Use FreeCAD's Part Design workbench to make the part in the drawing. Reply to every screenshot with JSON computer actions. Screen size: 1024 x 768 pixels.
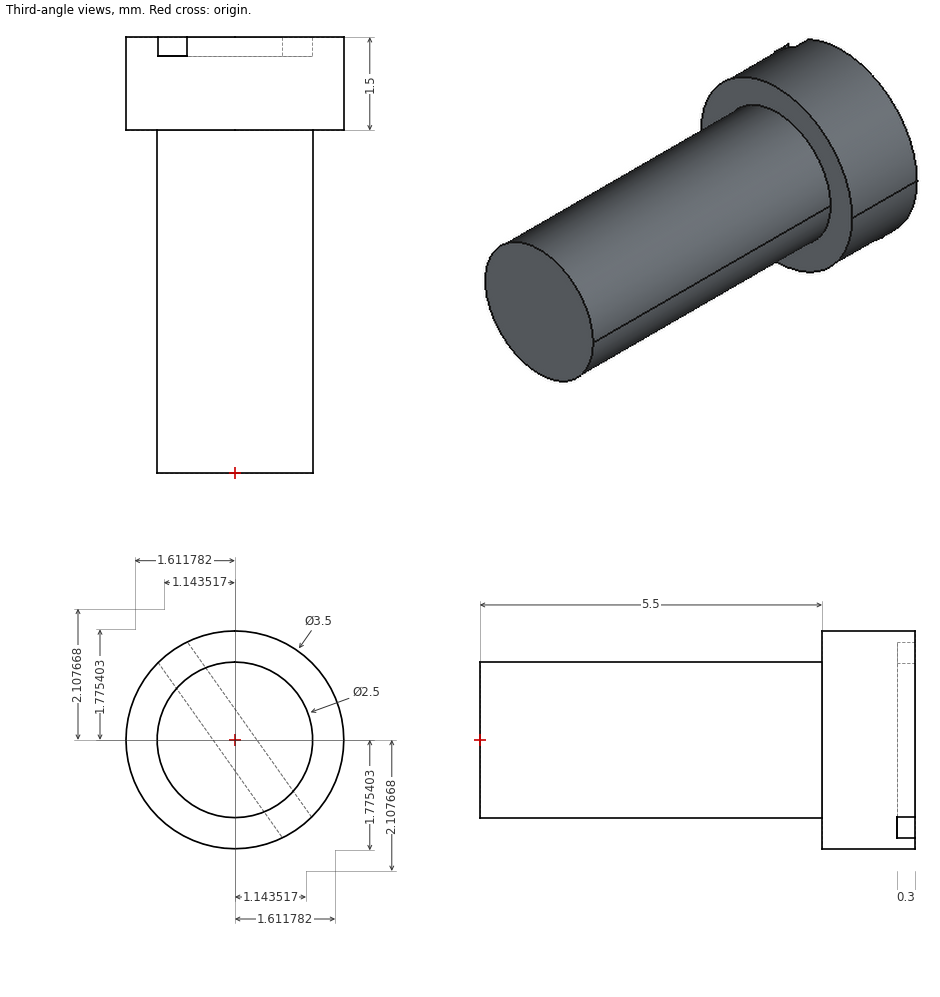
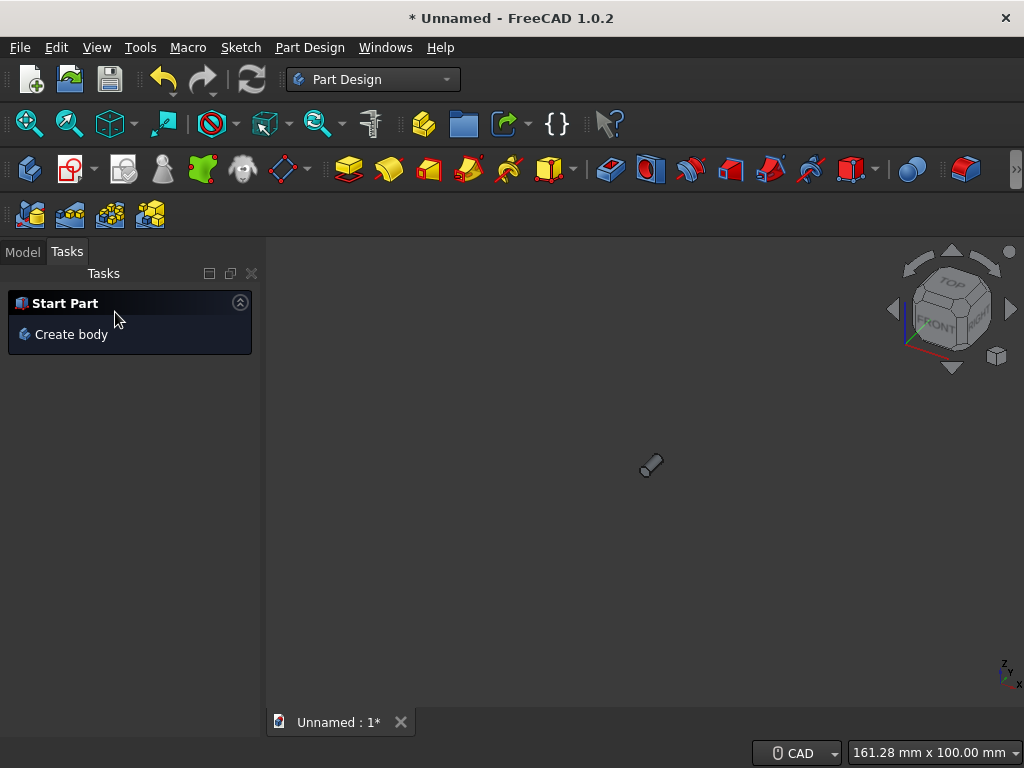
{"action": "key", "text": "v f"}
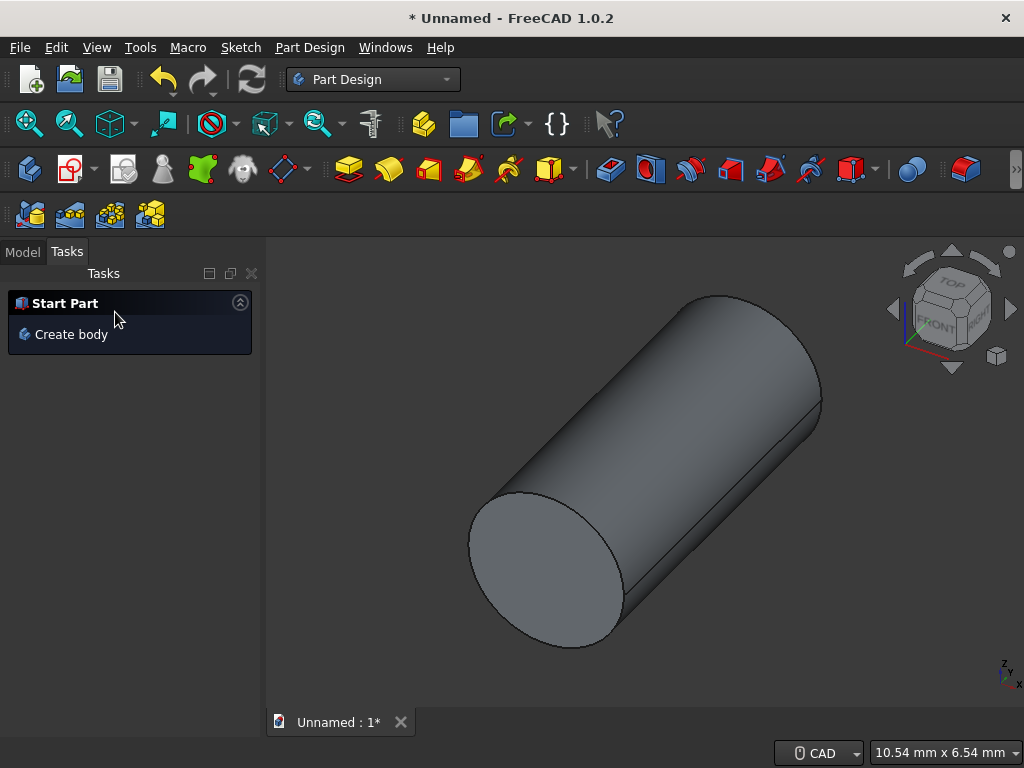
{"action": "key", "text": "4"}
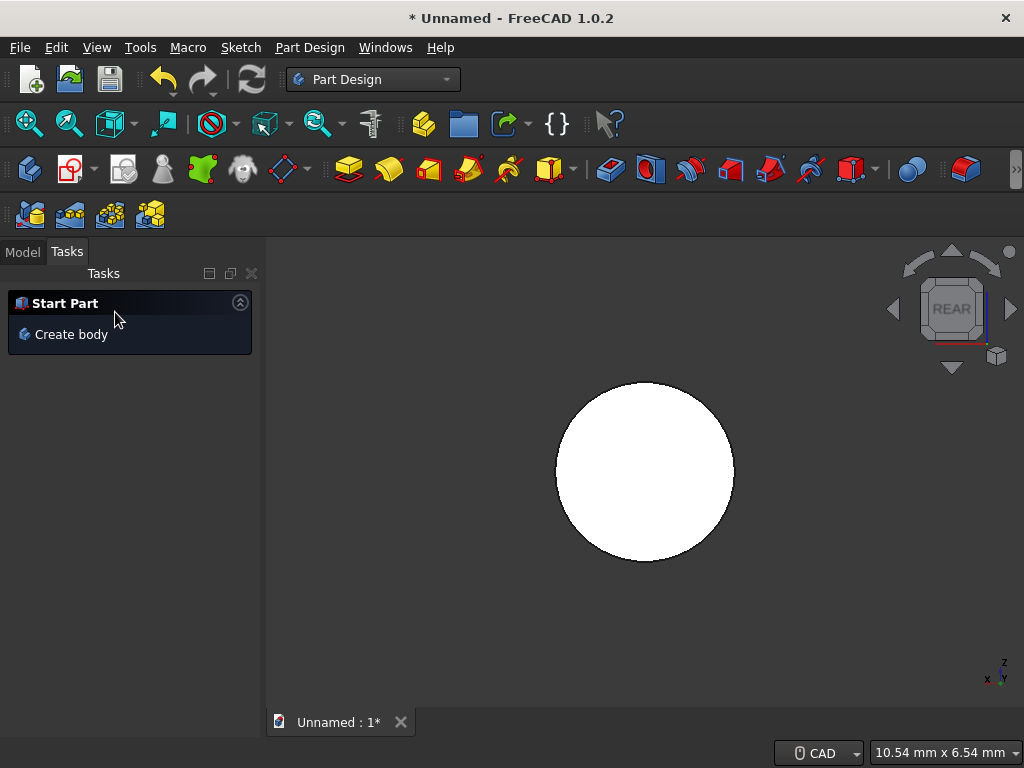
{"action": "left_click", "coordinate": [30, 124]}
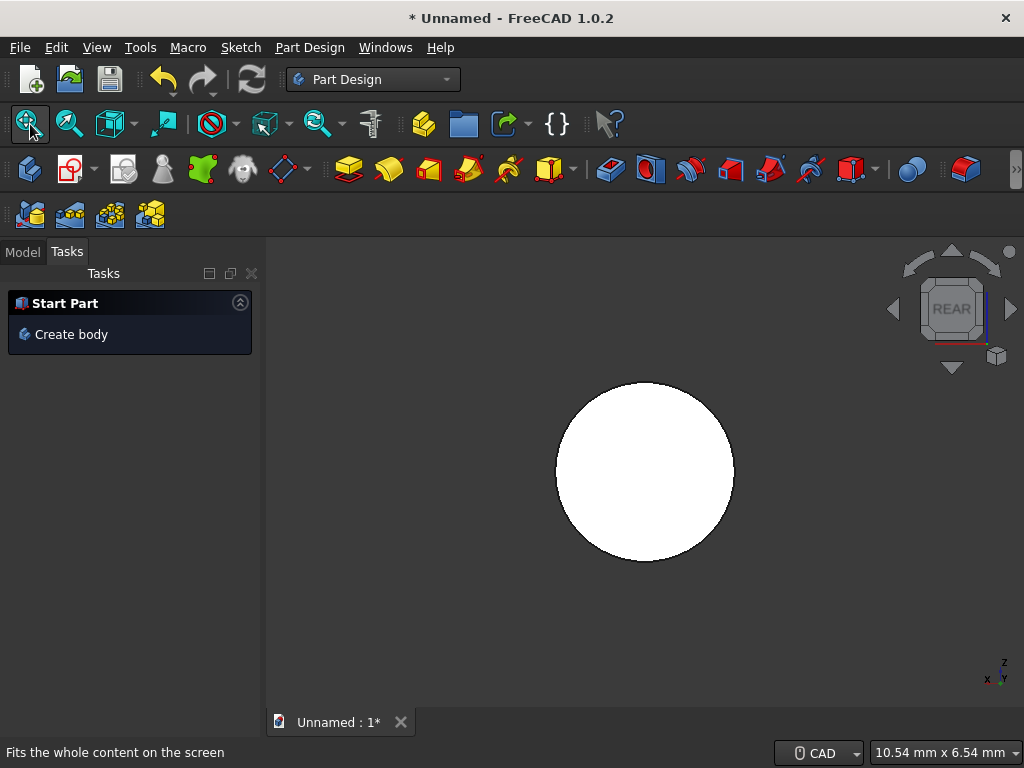
{"action": "left_click", "coordinate": [645, 471]}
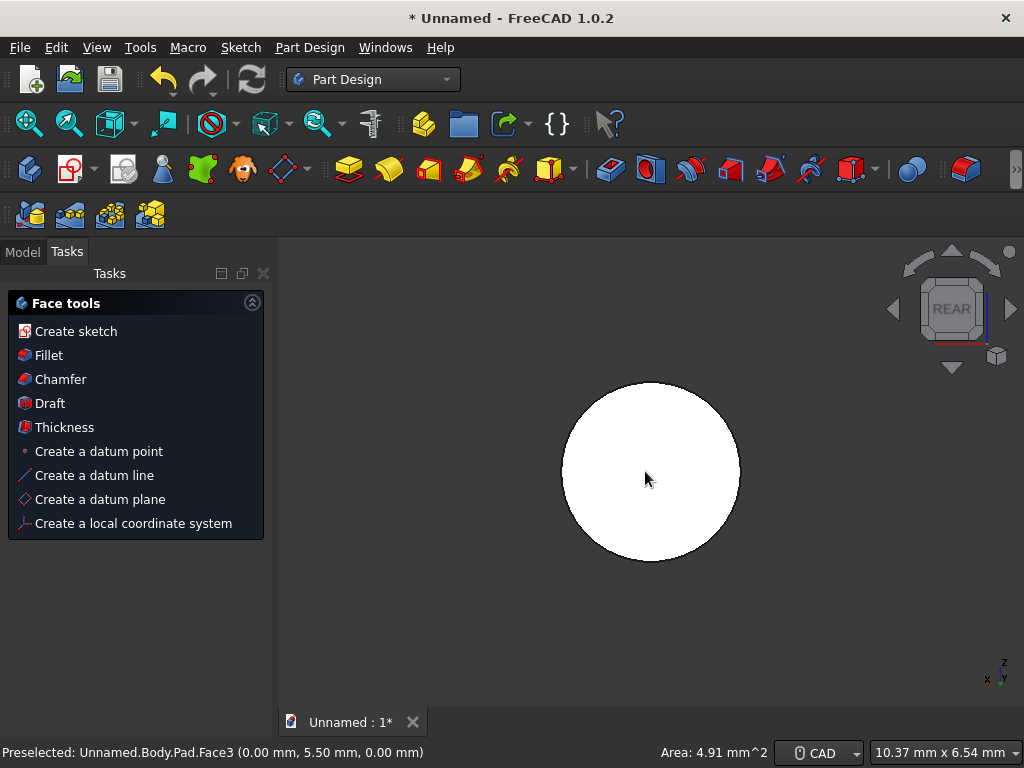
{"action": "left_click", "coordinate": [70, 170]}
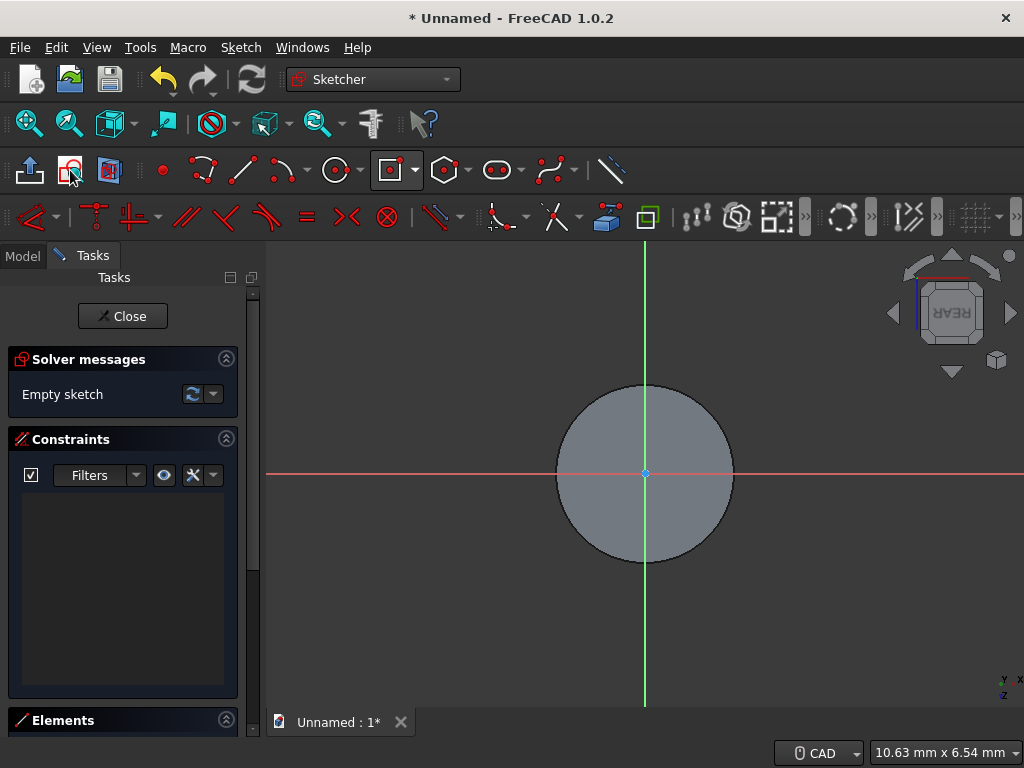
{"action": "key", "text": "g c"}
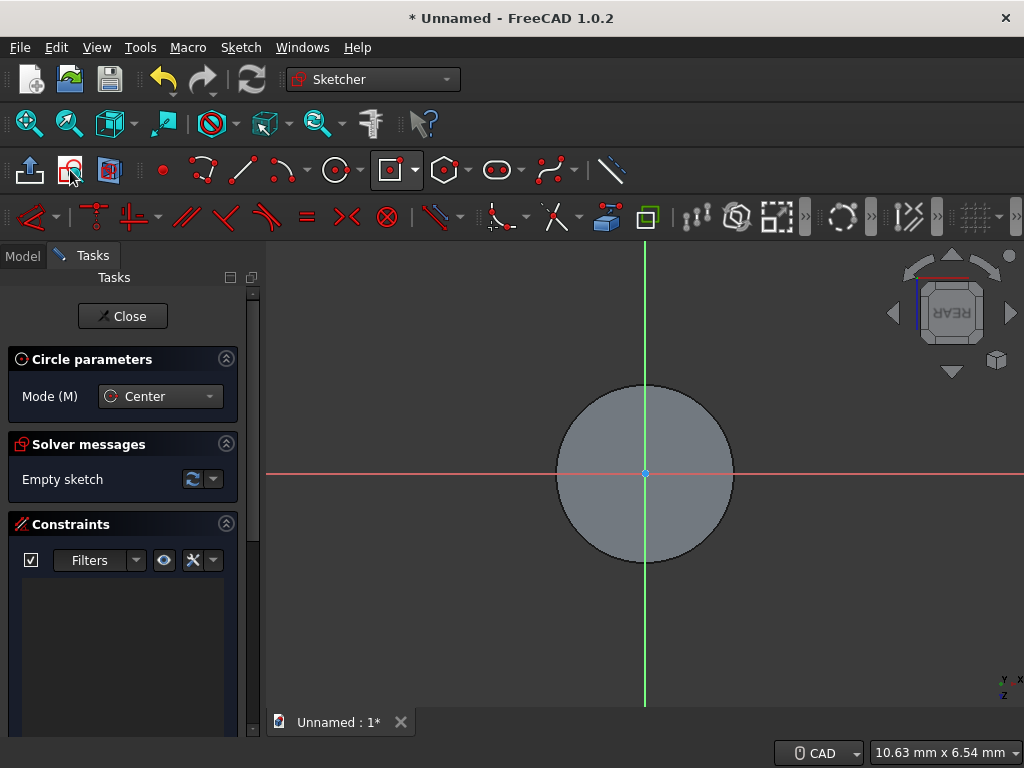
{"action": "left_click", "coordinate": [645, 474]}
{"action": "mouse_move", "coordinate": [733, 386]}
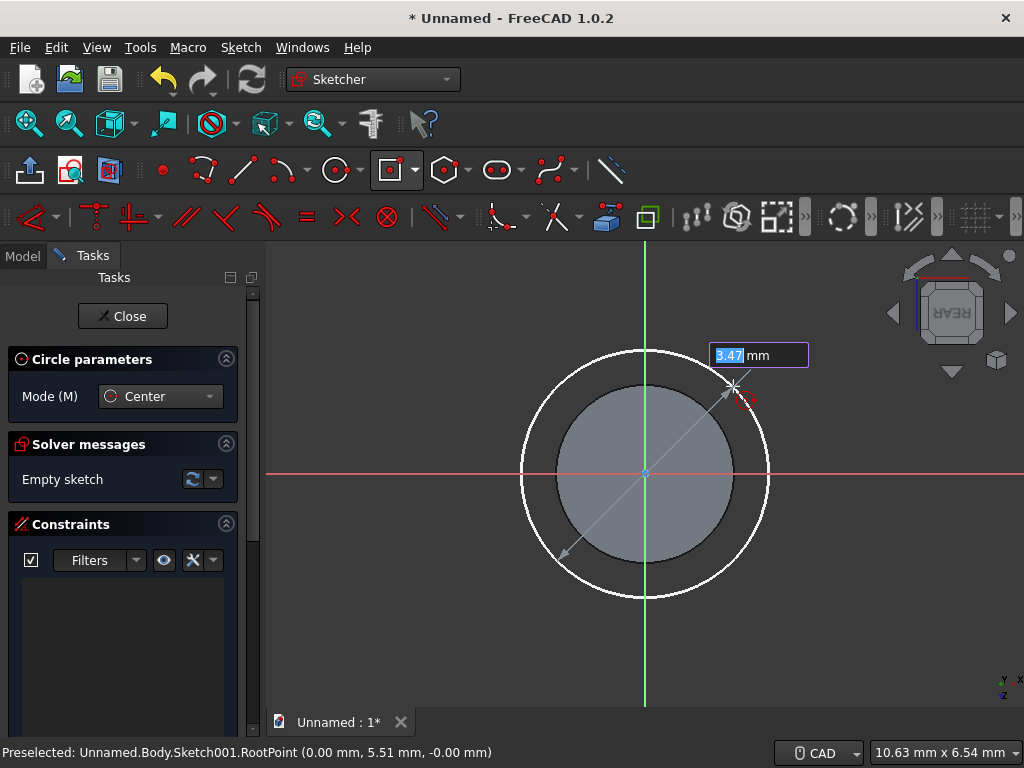
{"action": "type", "text": "3.5"}
{"action": "key", "text": "Return"}
{"action": "key", "text": "Escape"}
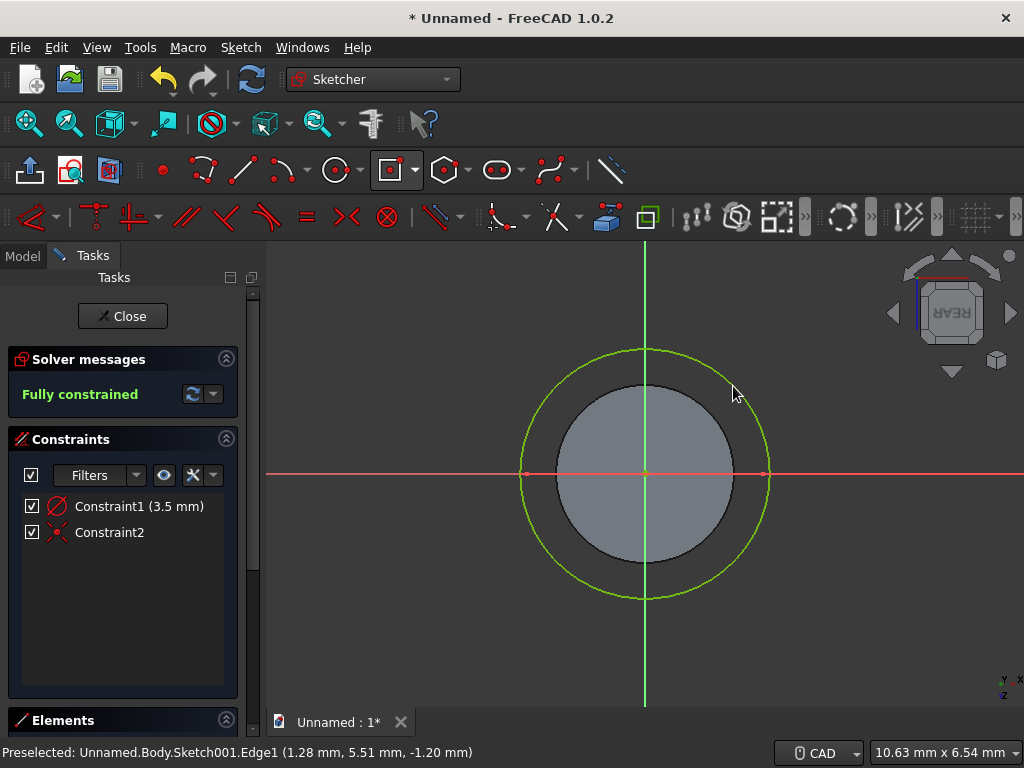
{"action": "left_click", "coordinate": [123, 316]}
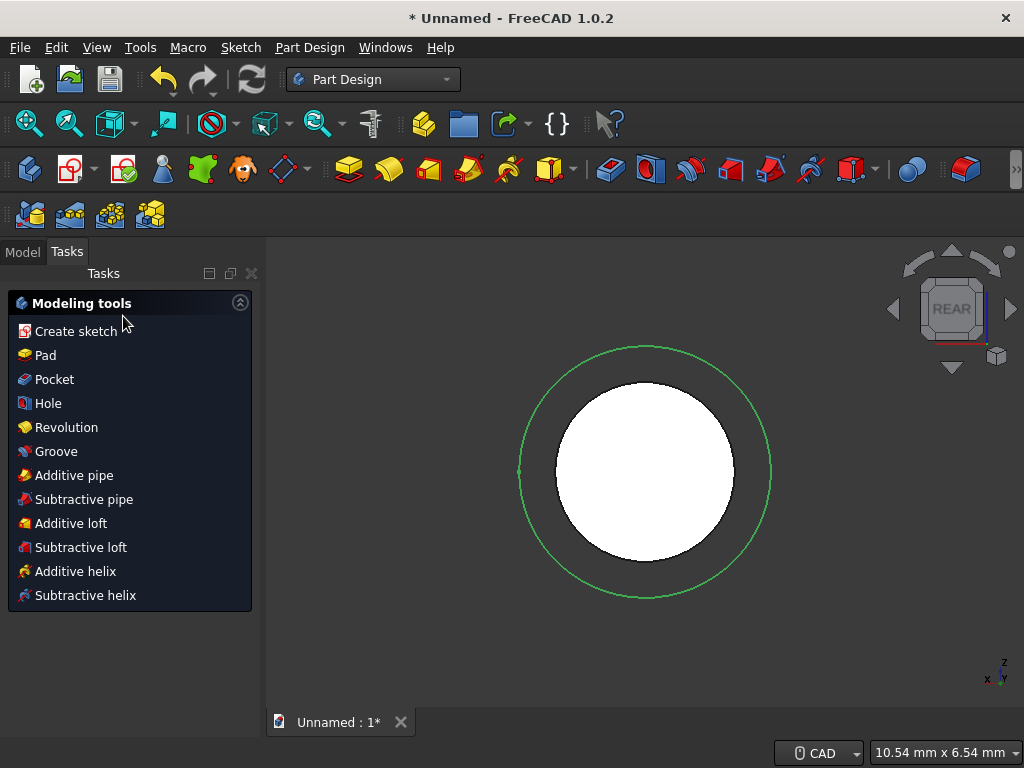
{"action": "left_click", "coordinate": [350, 170]}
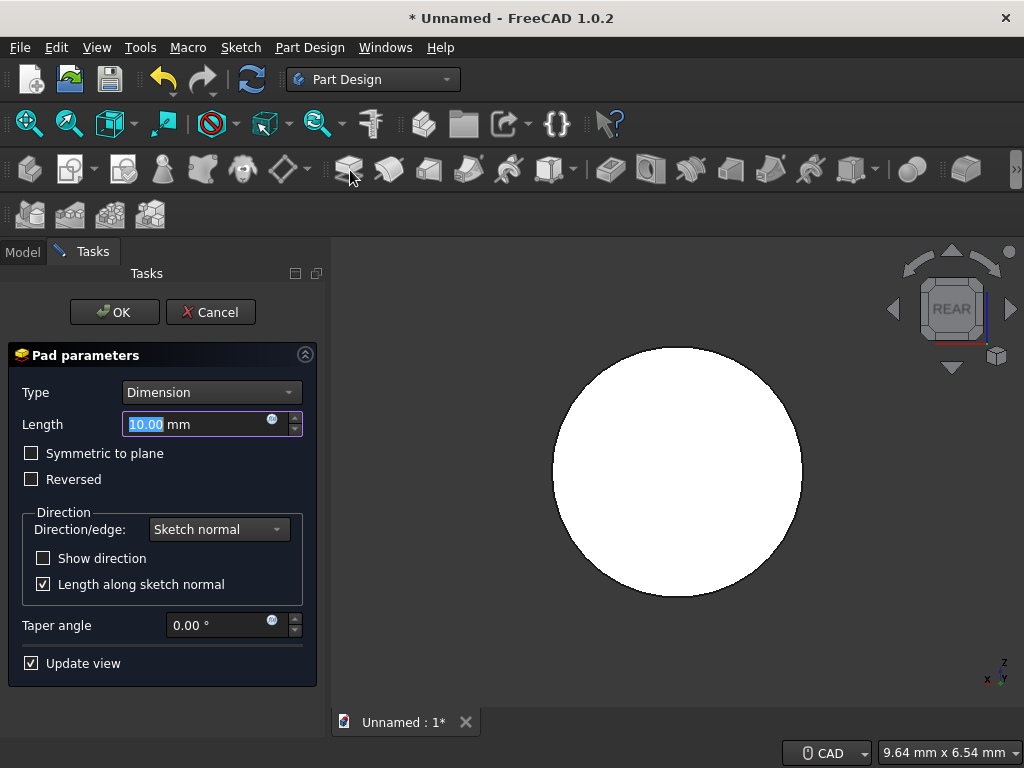
{"action": "type", "text": "1.5"}
{"action": "key", "text": "Tab"}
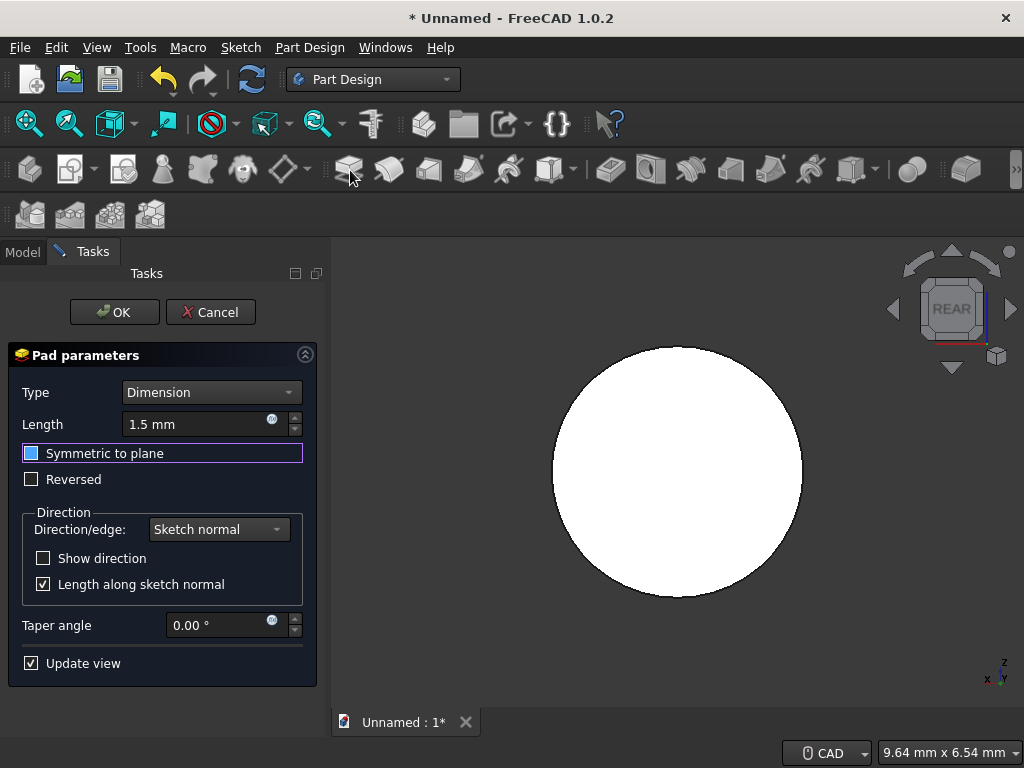
{"action": "left_click", "coordinate": [115, 312]}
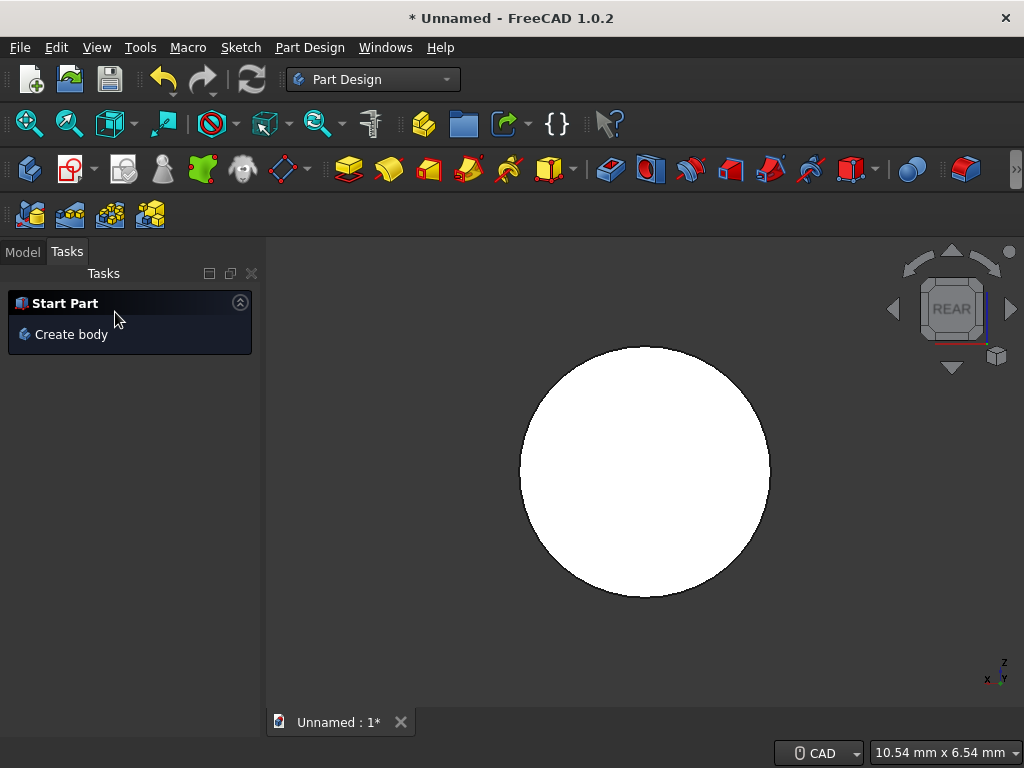
{"action": "left_click", "coordinate": [645, 471]}